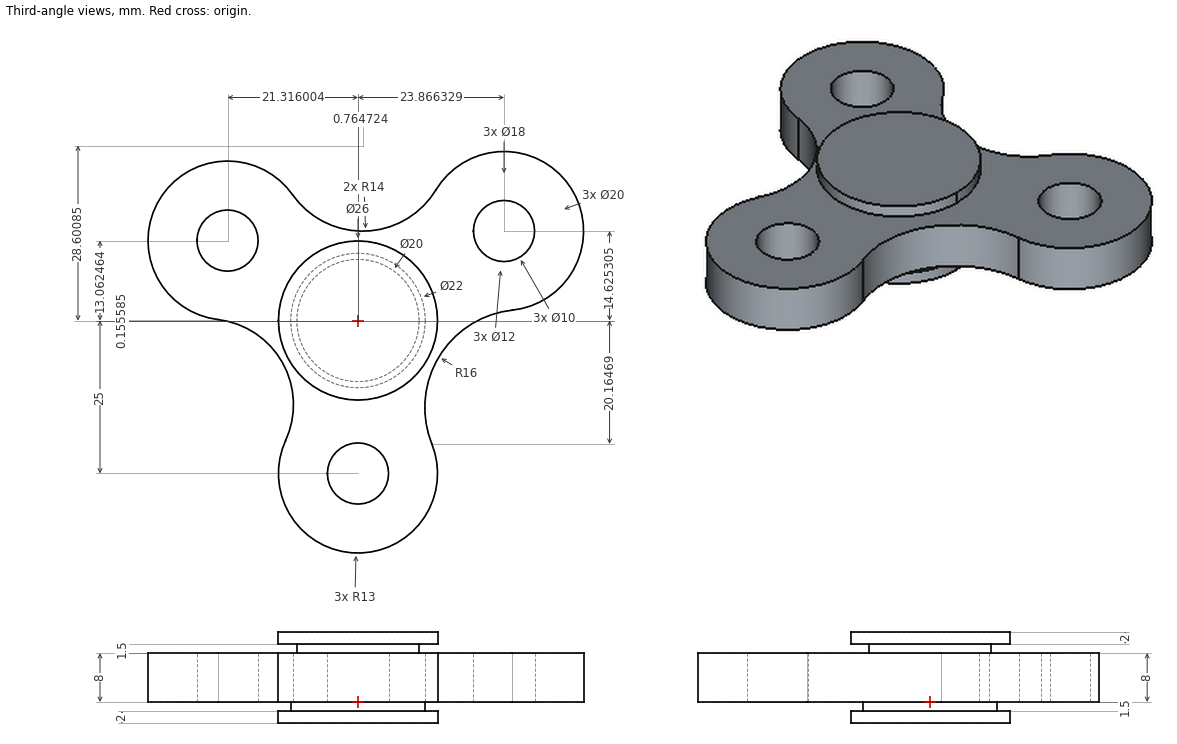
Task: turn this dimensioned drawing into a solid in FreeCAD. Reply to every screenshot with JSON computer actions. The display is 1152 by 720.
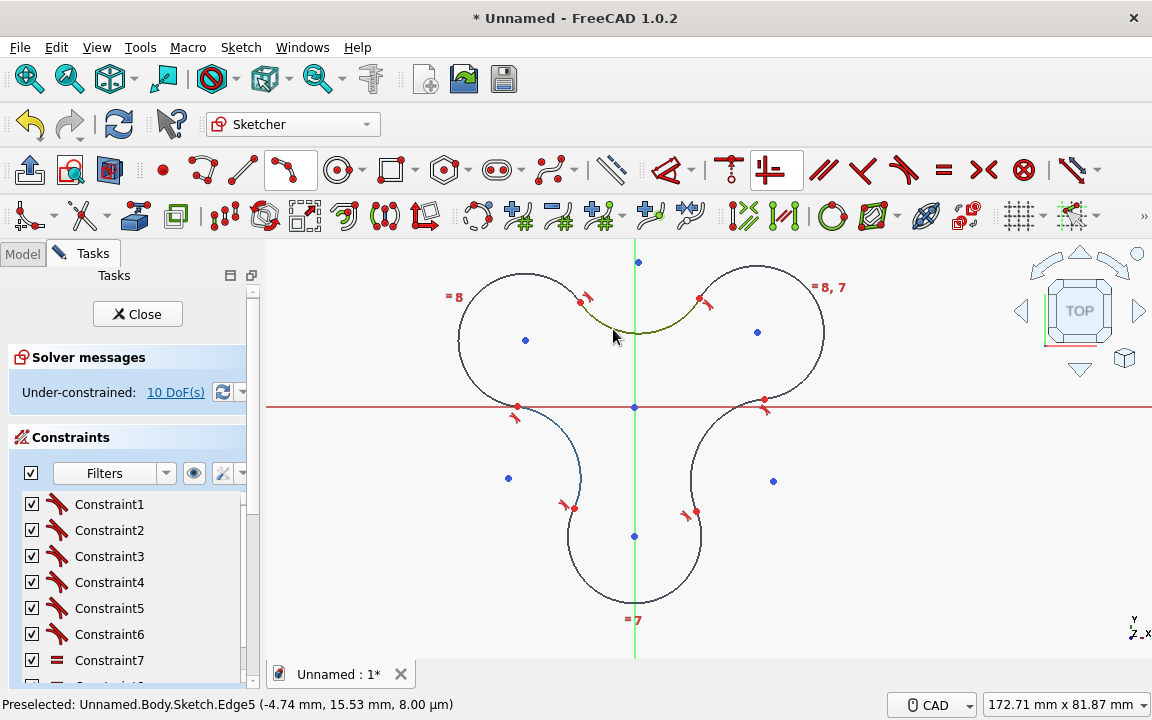
{"action": "left_click", "coordinate": [944, 170]}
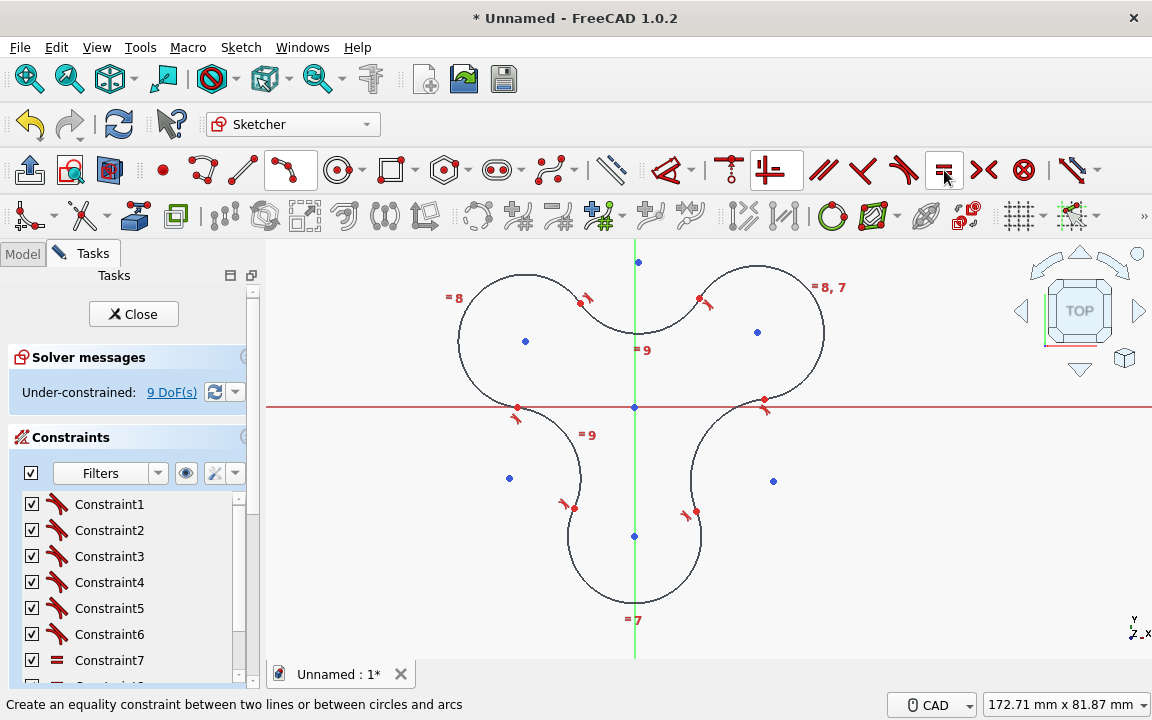
{"action": "left_click", "coordinate": [635, 537]}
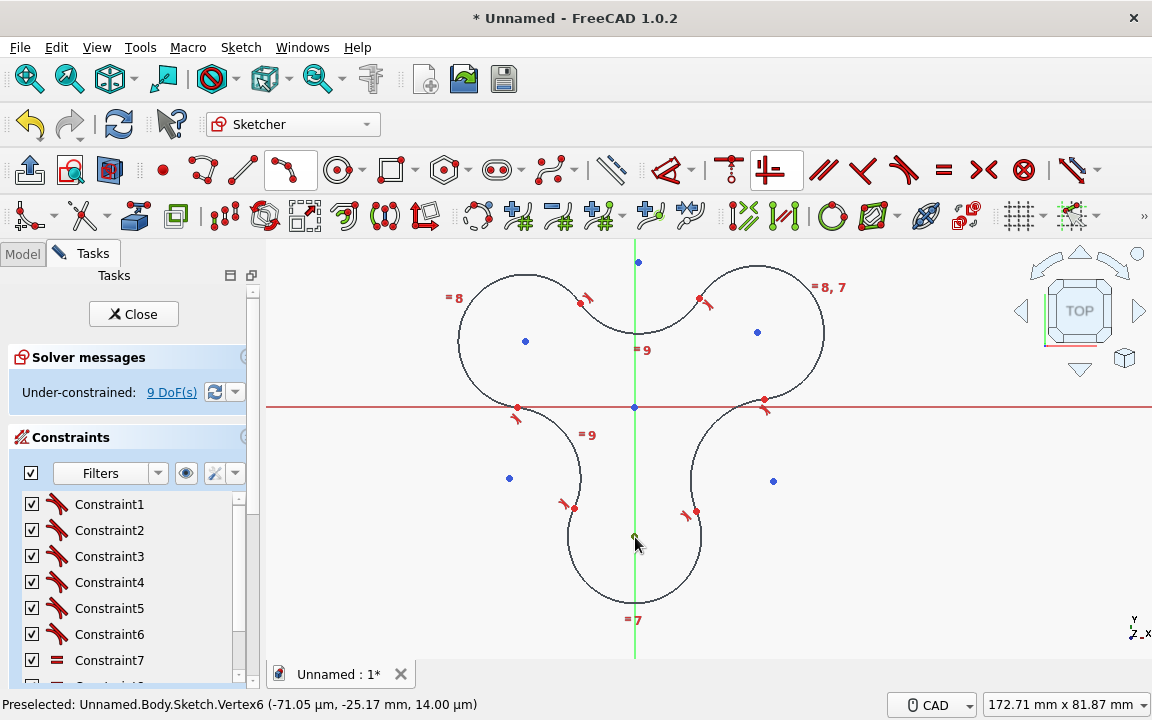
{"action": "left_click", "coordinate": [635, 553]}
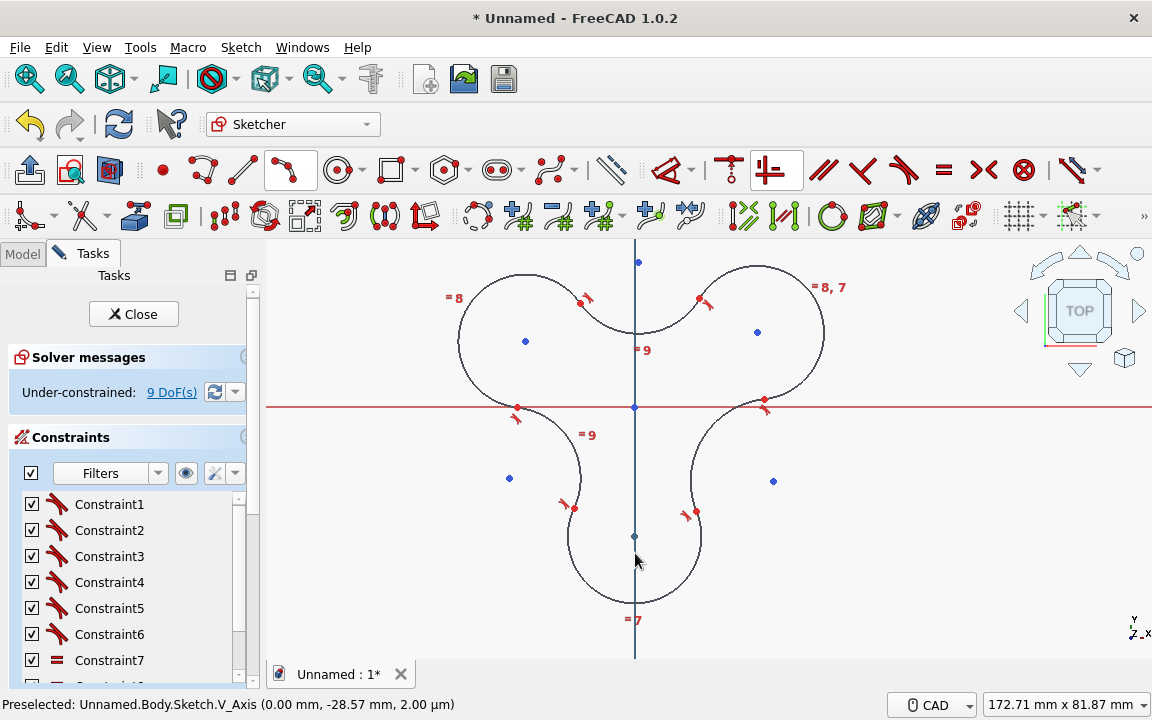
{"action": "left_click", "coordinate": [730, 170]}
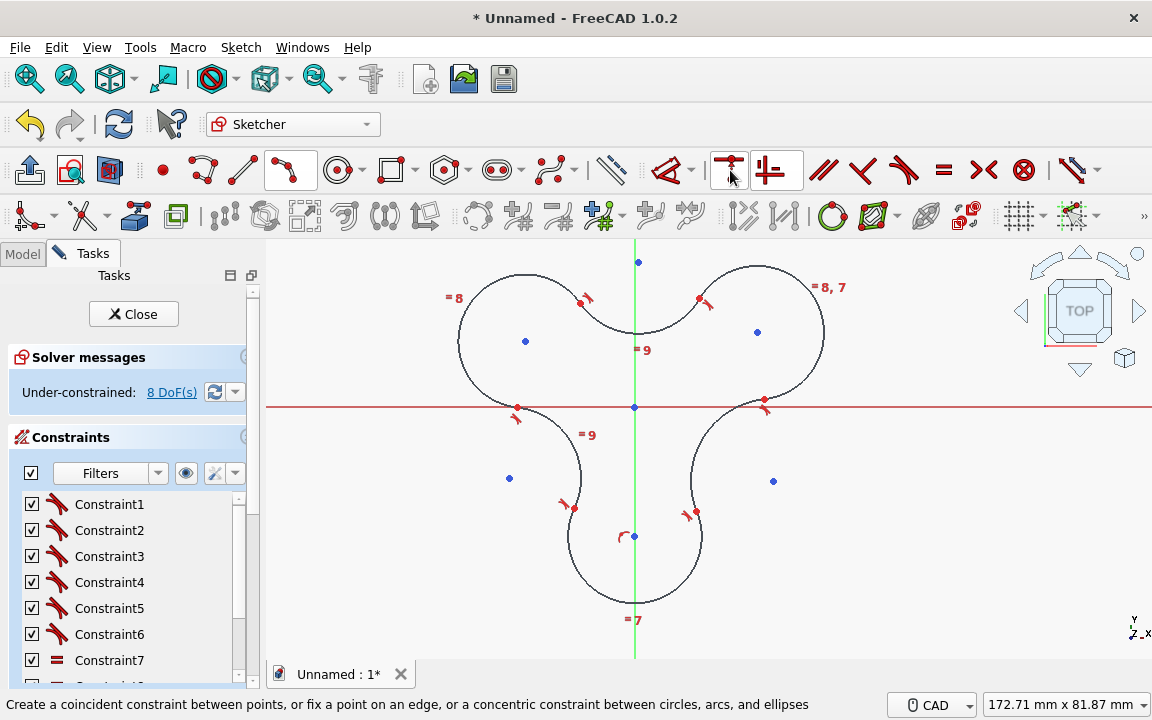
{"action": "left_click", "coordinate": [580, 469]}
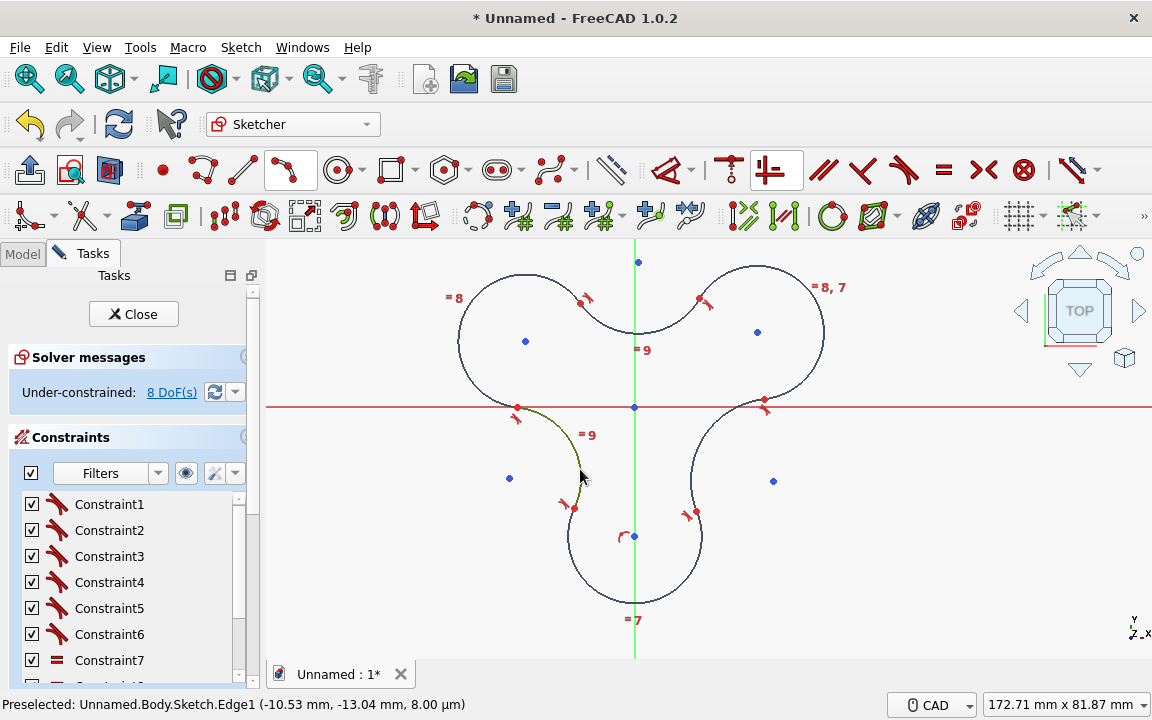
{"action": "left_click", "coordinate": [694, 170]}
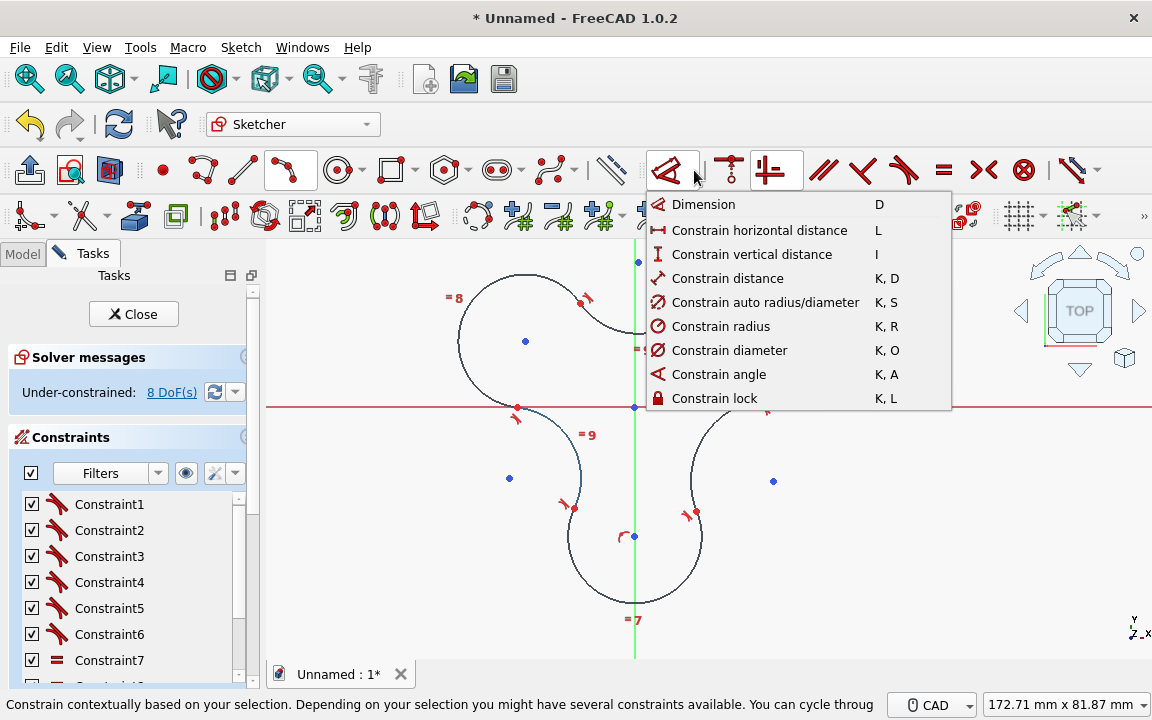
{"action": "left_click", "coordinate": [799, 326]}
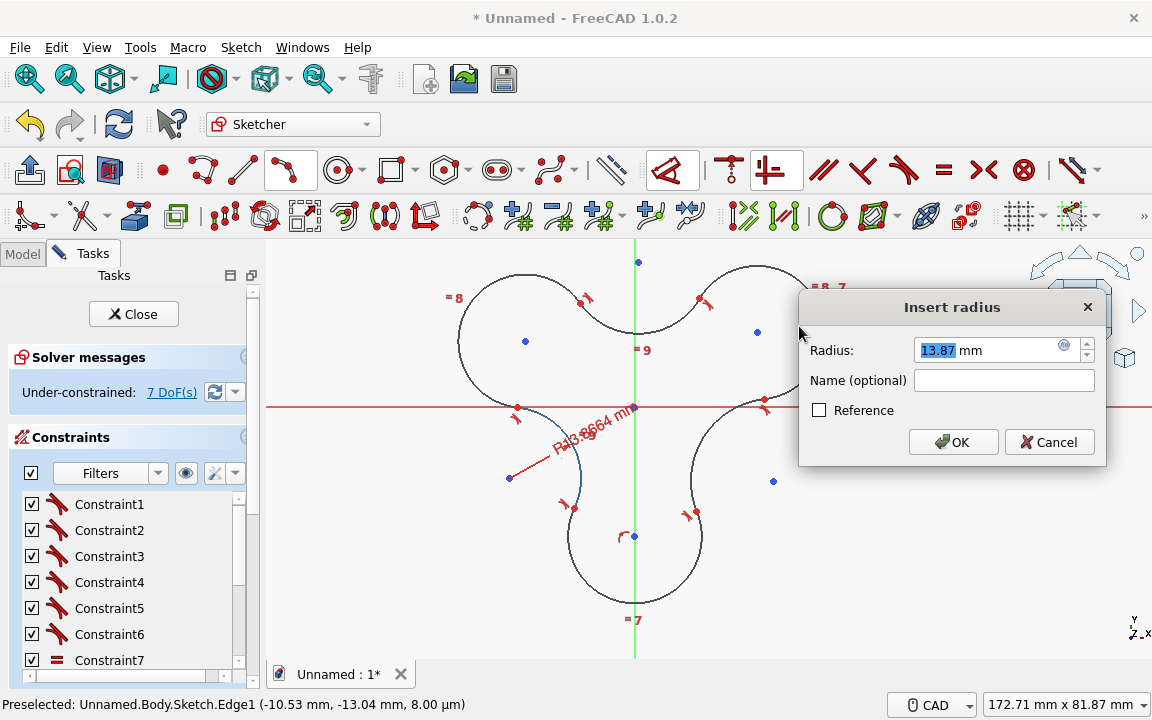
{"action": "type", "text": "14"}
{"action": "key", "text": "Return"}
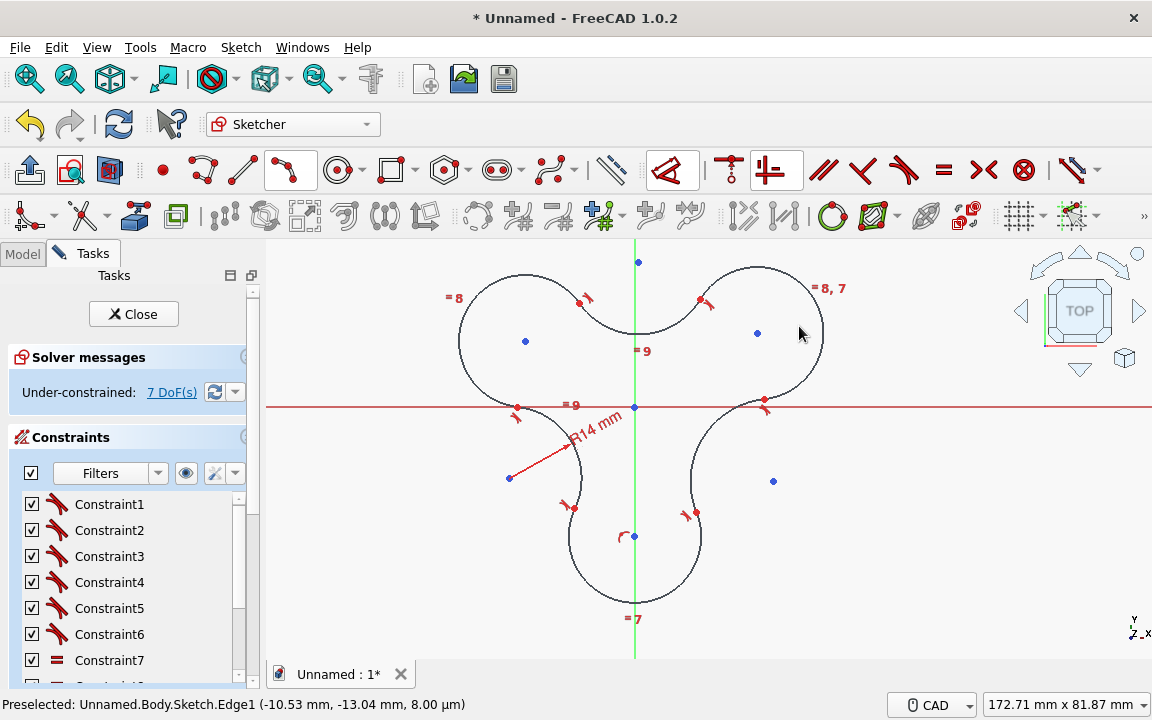
{"action": "left_click", "coordinate": [587, 582]}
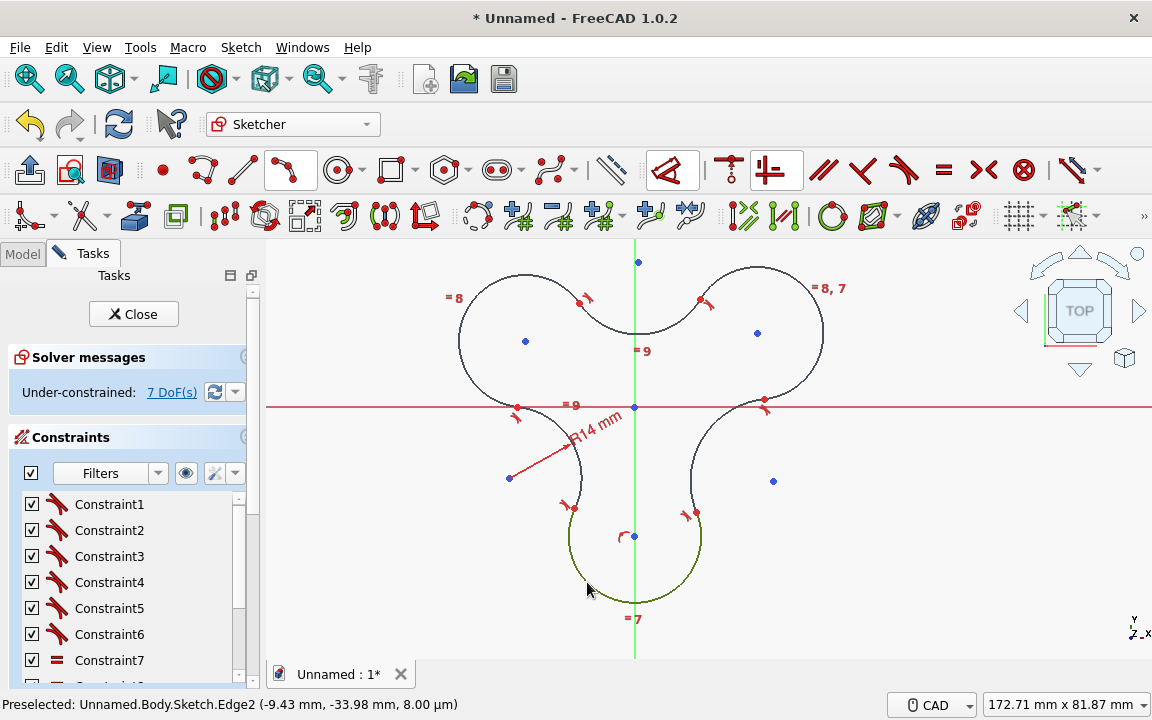
{"action": "key", "text": "k r"}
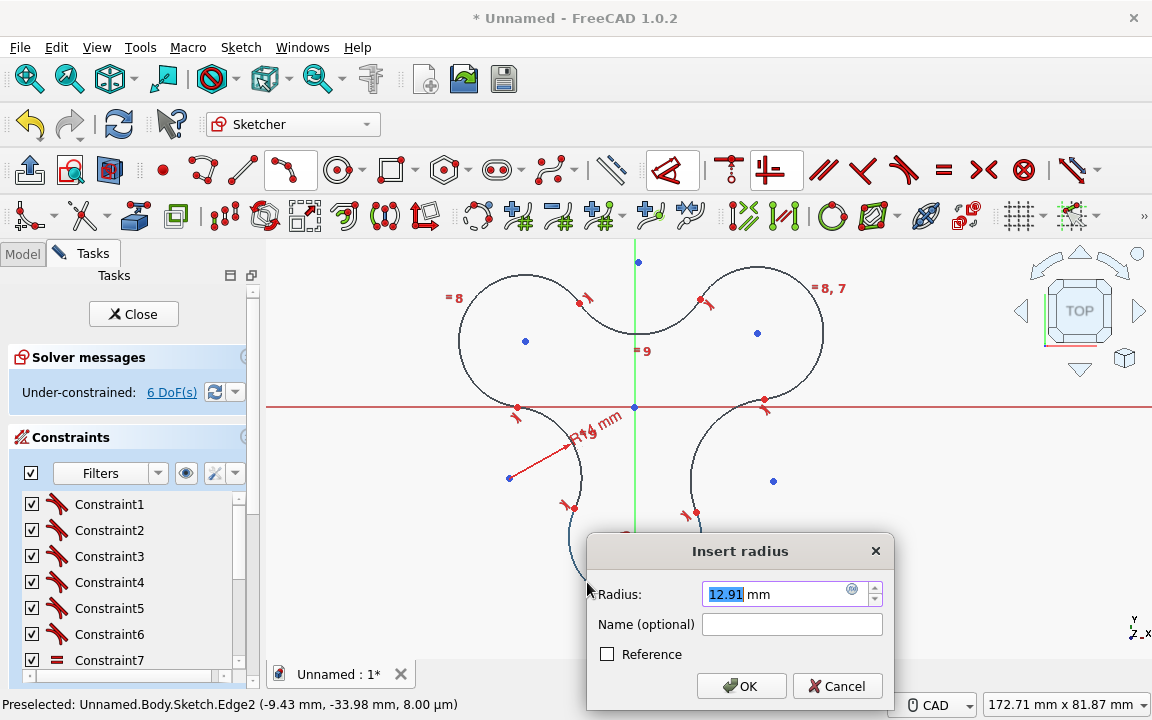
{"action": "type", "text": "13"}
{"action": "key", "text": "Return"}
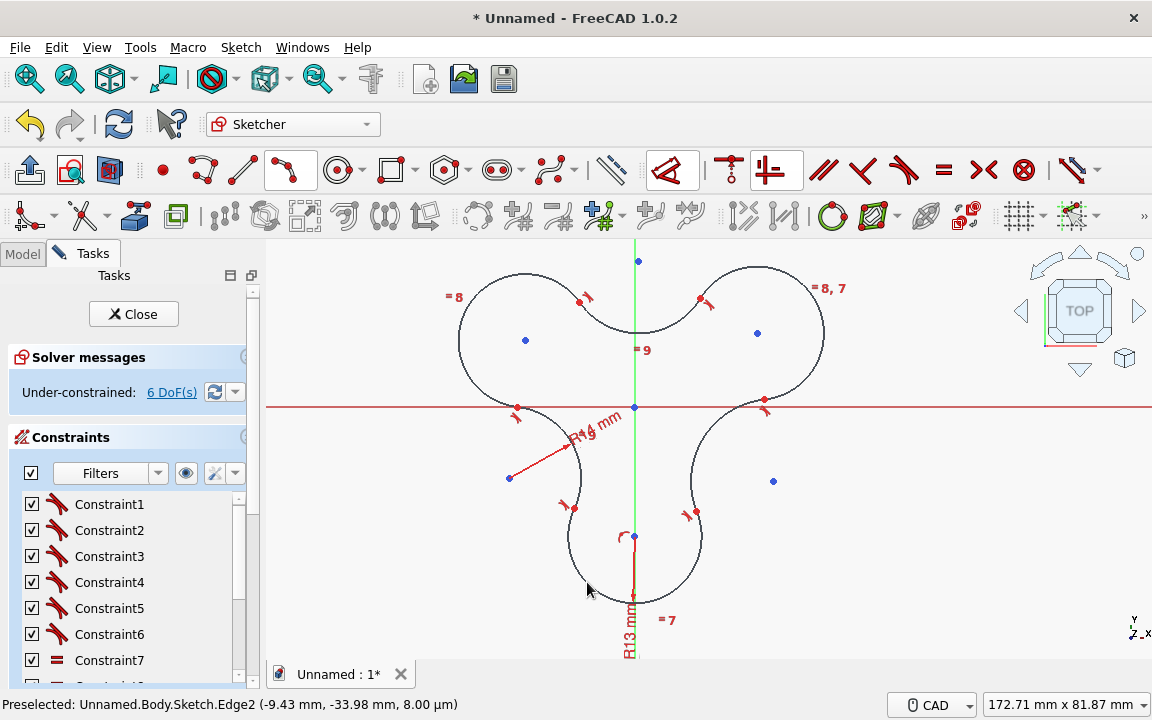
{"action": "scroll", "coordinate": [723, 416], "scroll_direction": "up", "scroll_amount": 3}